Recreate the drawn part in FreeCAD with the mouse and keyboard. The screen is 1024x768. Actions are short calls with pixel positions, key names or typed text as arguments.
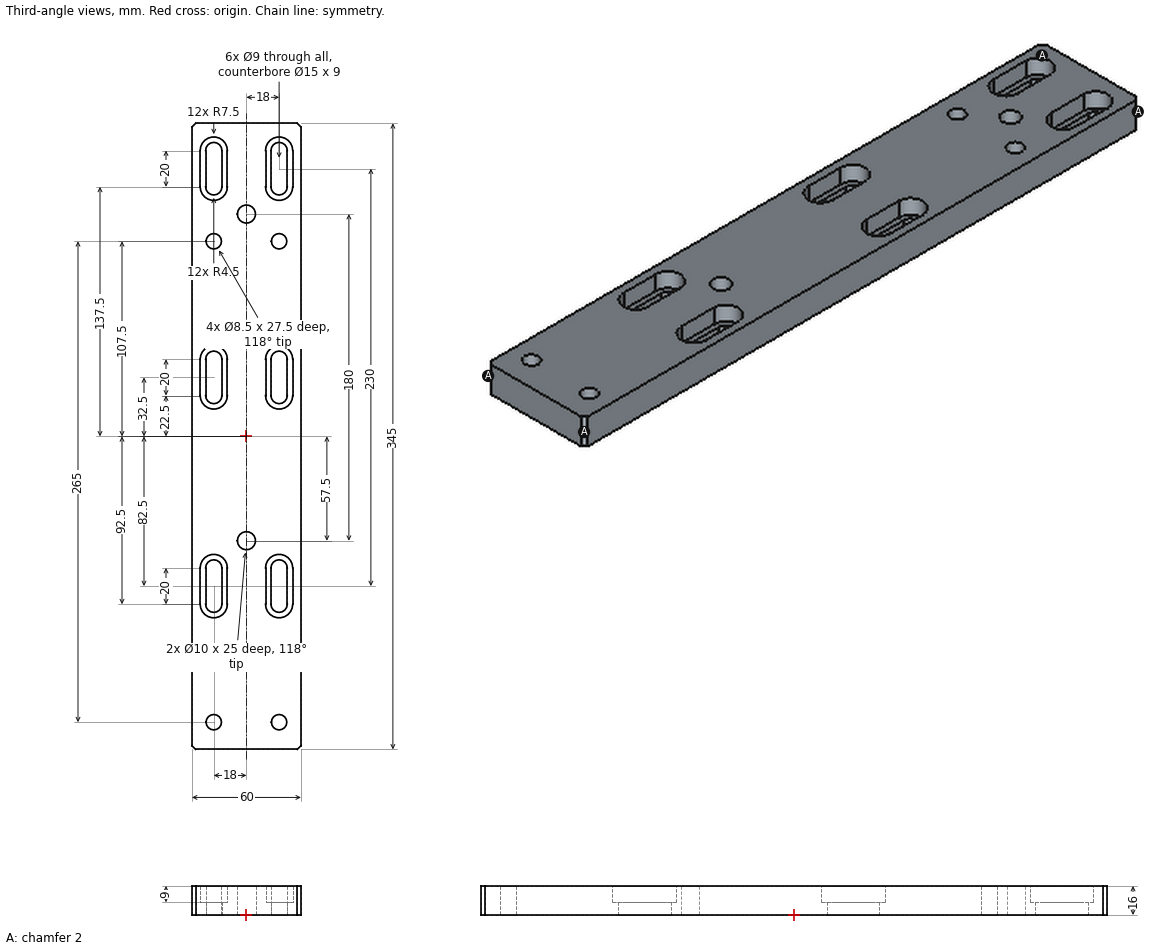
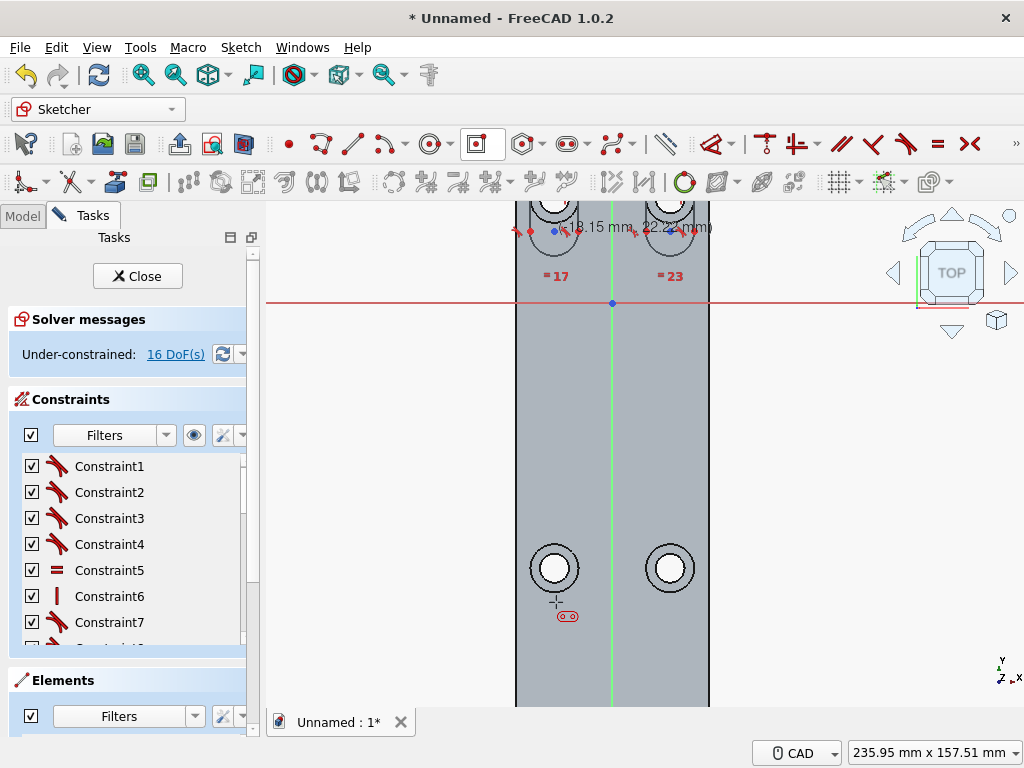
click(554, 600)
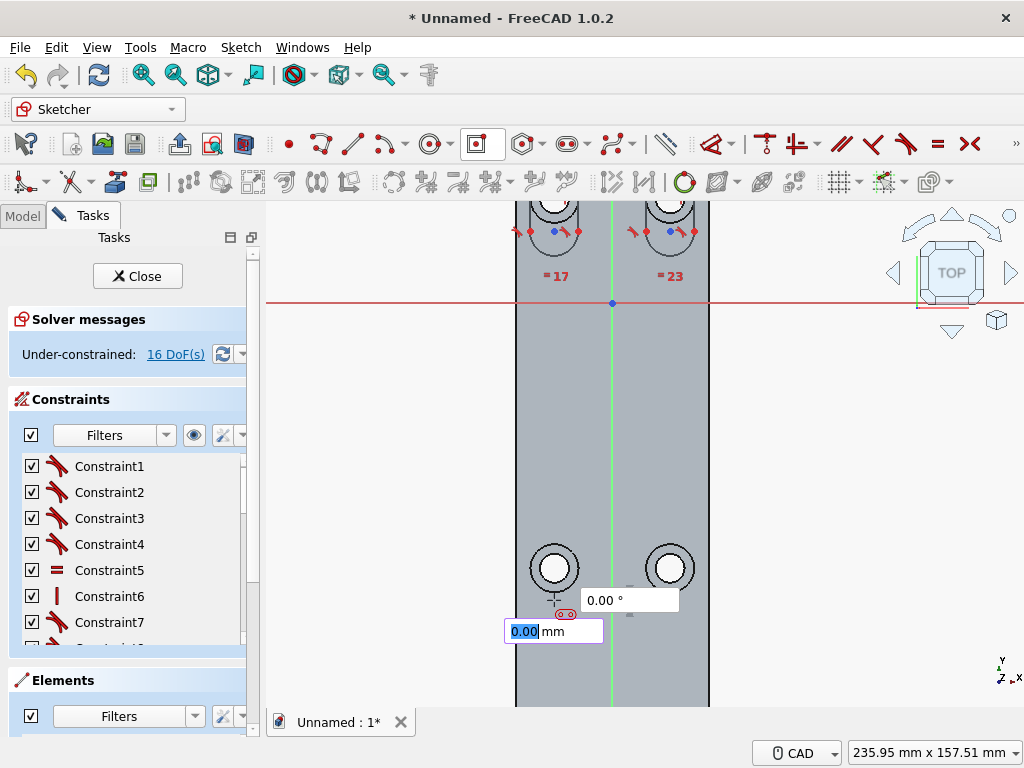
click(554, 536)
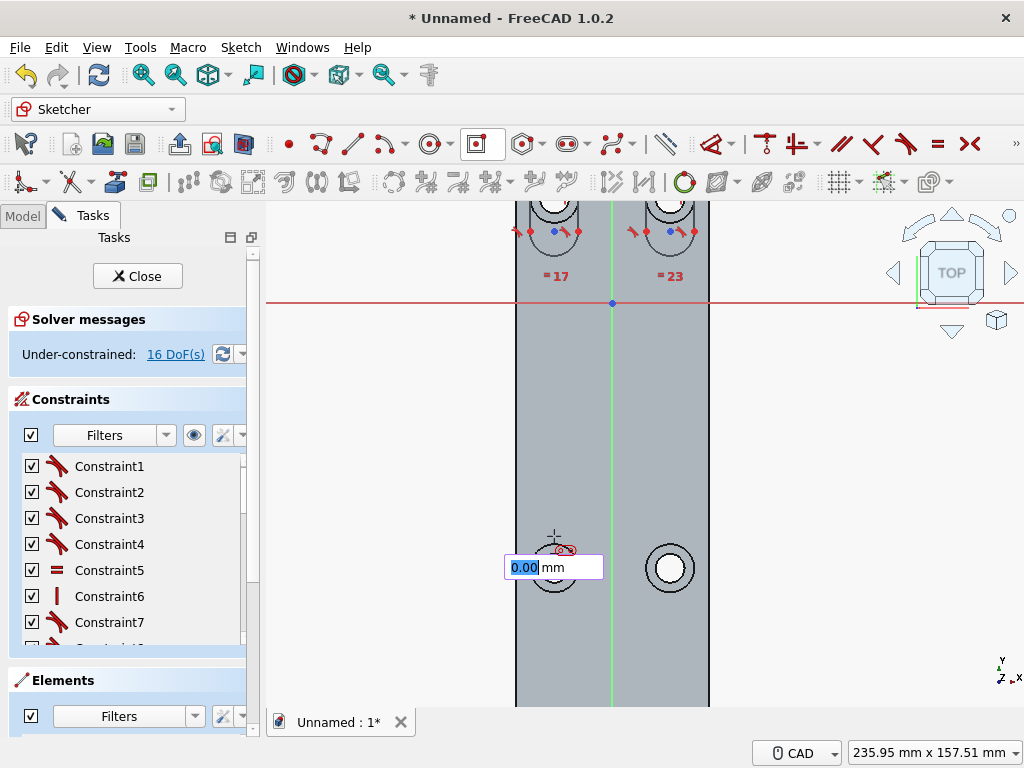
click(530, 568)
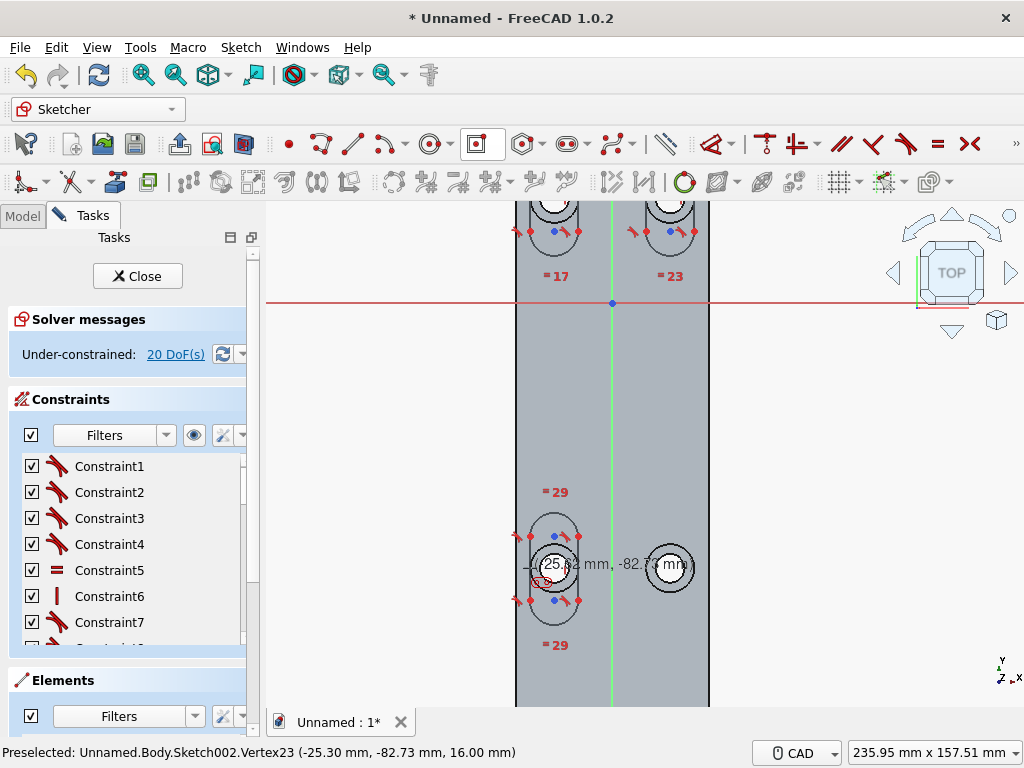
click(670, 600)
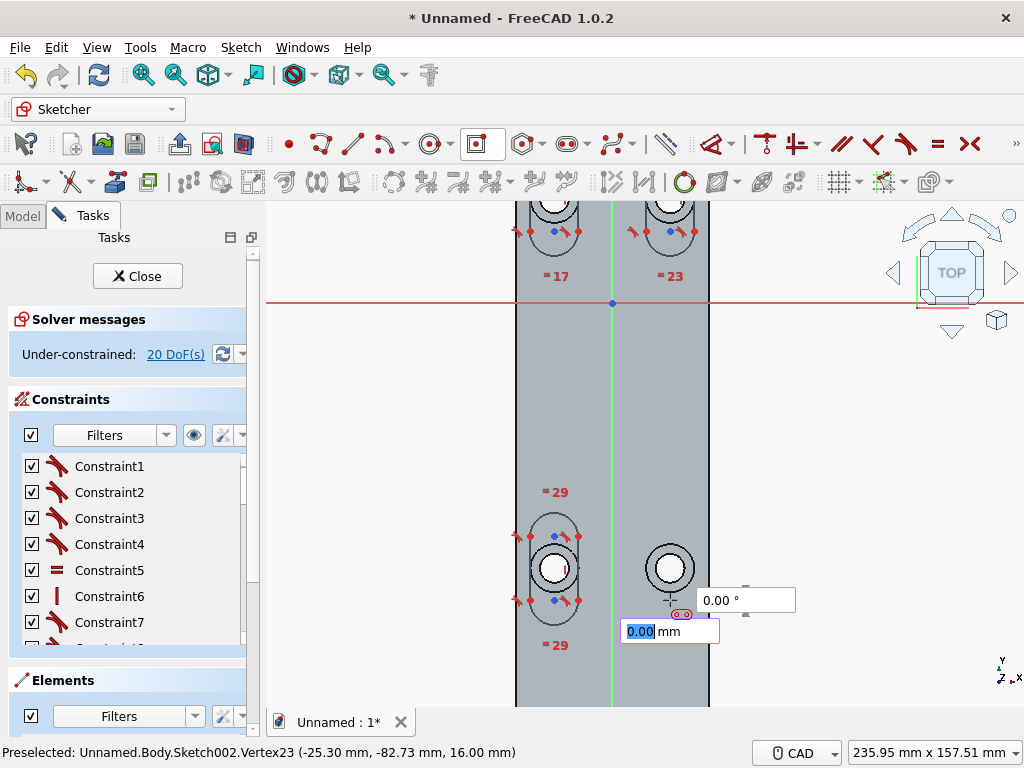
click(670, 536)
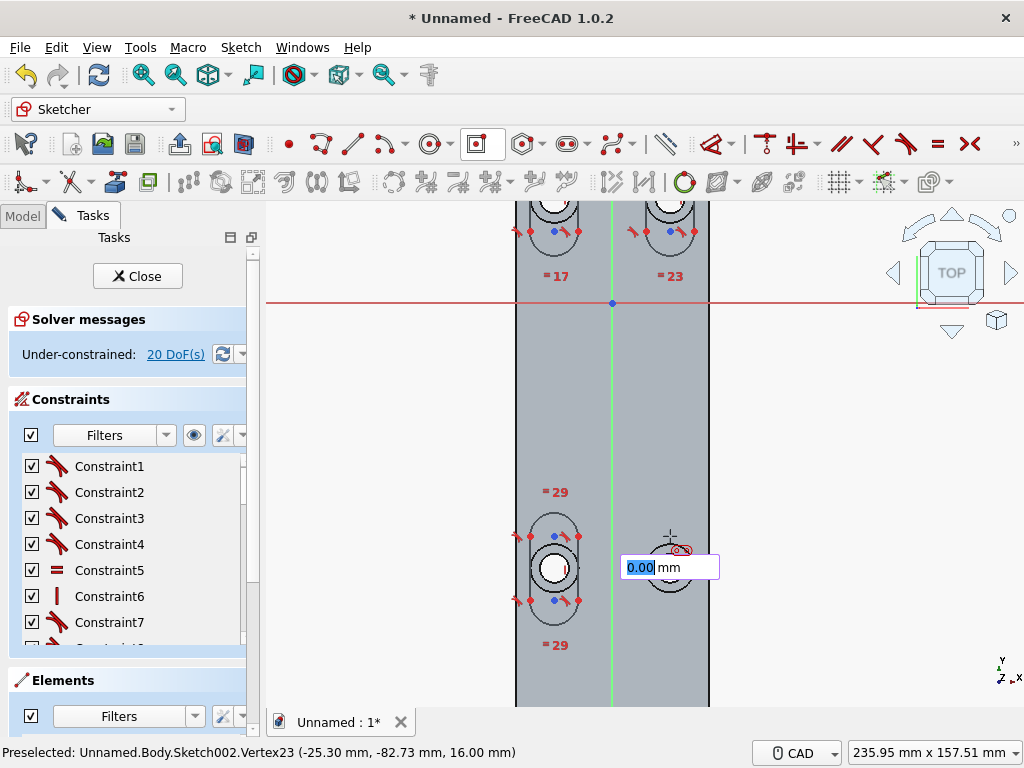
click(646, 568)
key(Escape)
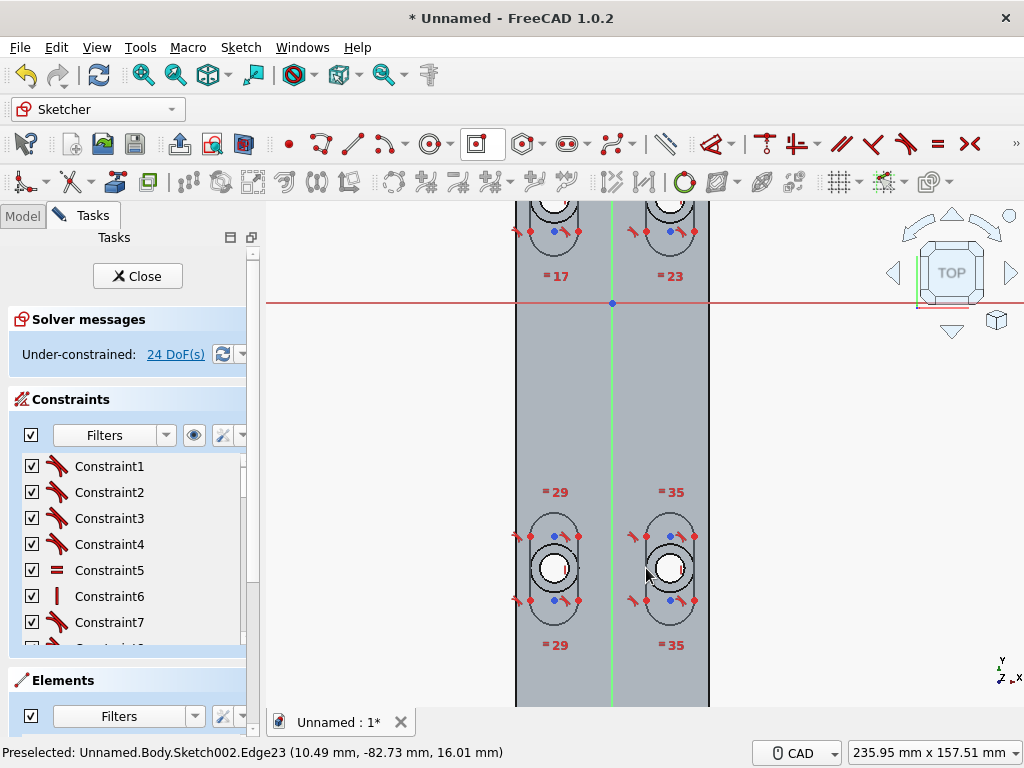
scroll(556, 602, down, 5)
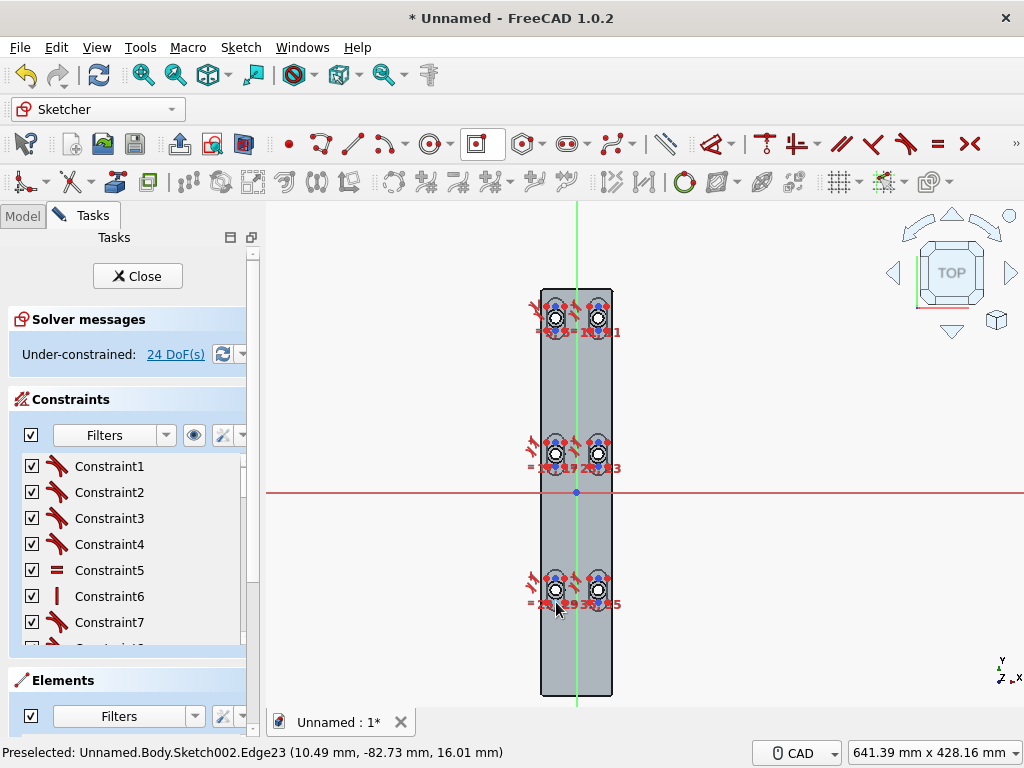
scroll(551, 338, up, 3)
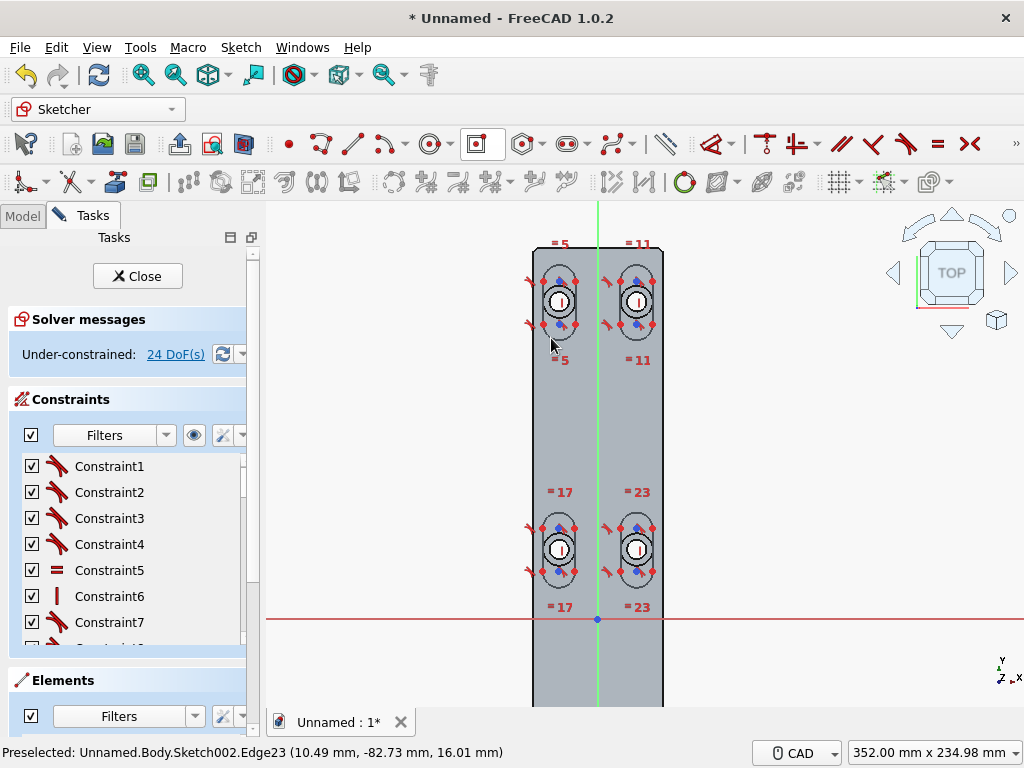
click(550, 337)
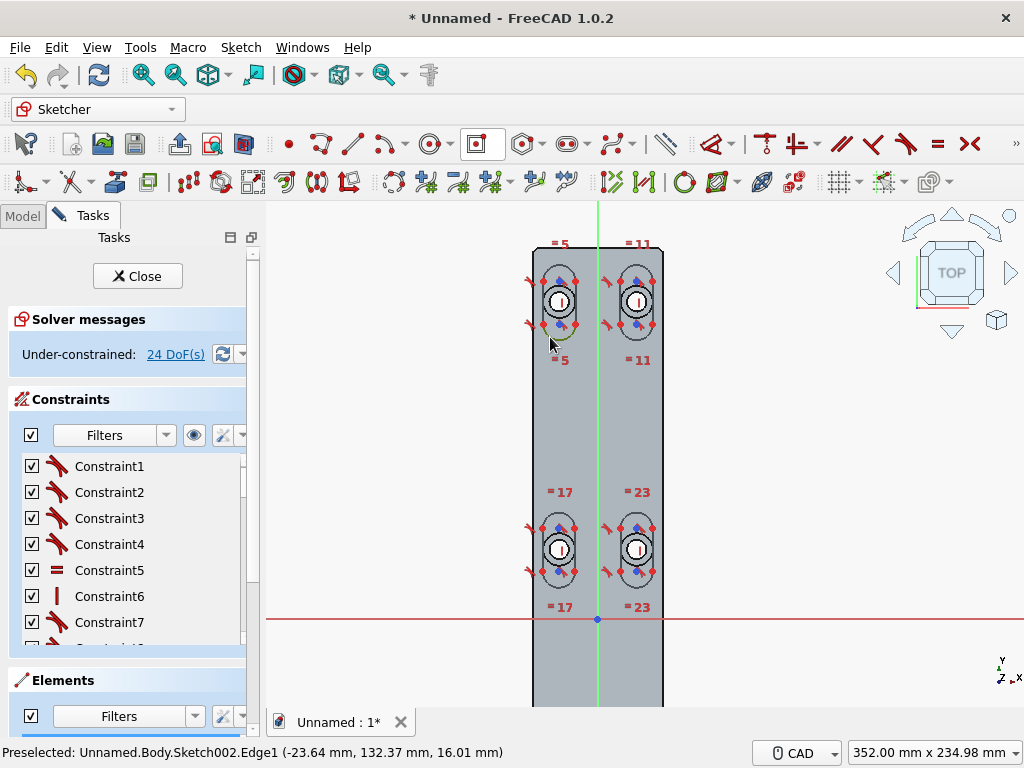
click(627, 337)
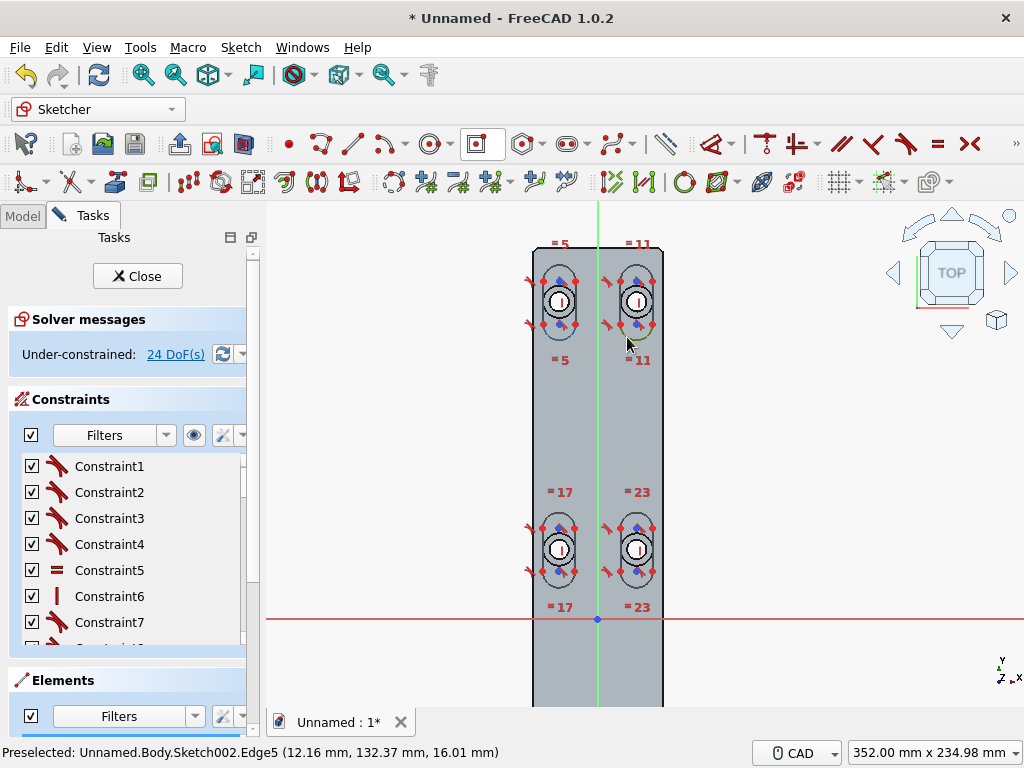
click(549, 585)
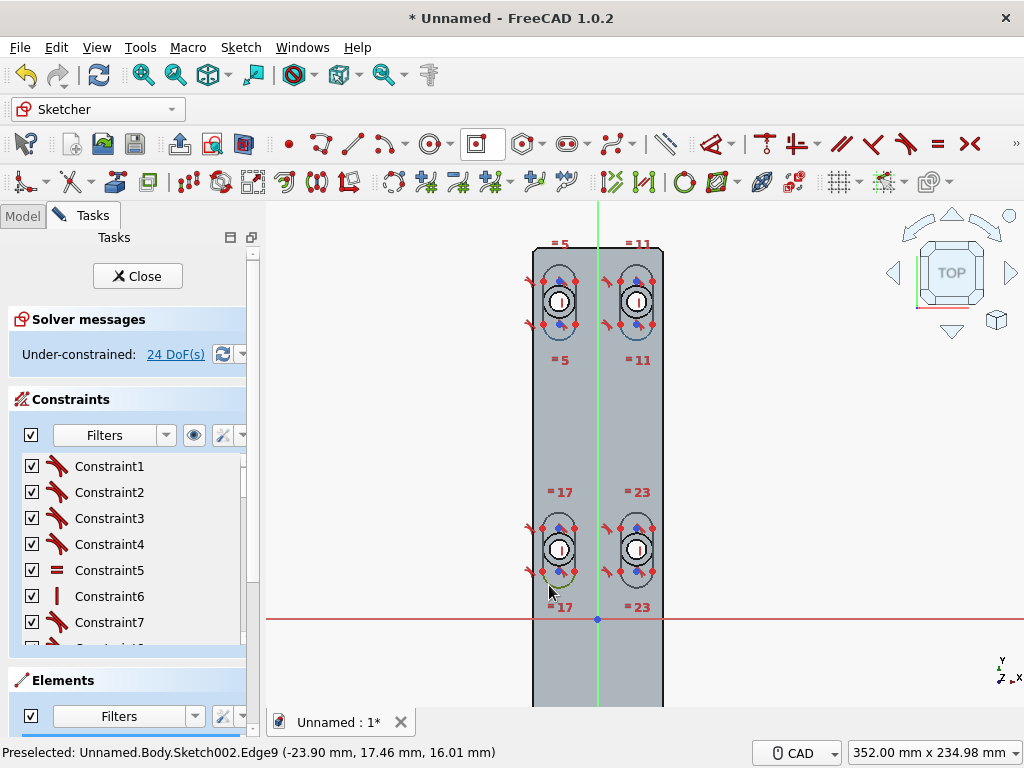
click(627, 585)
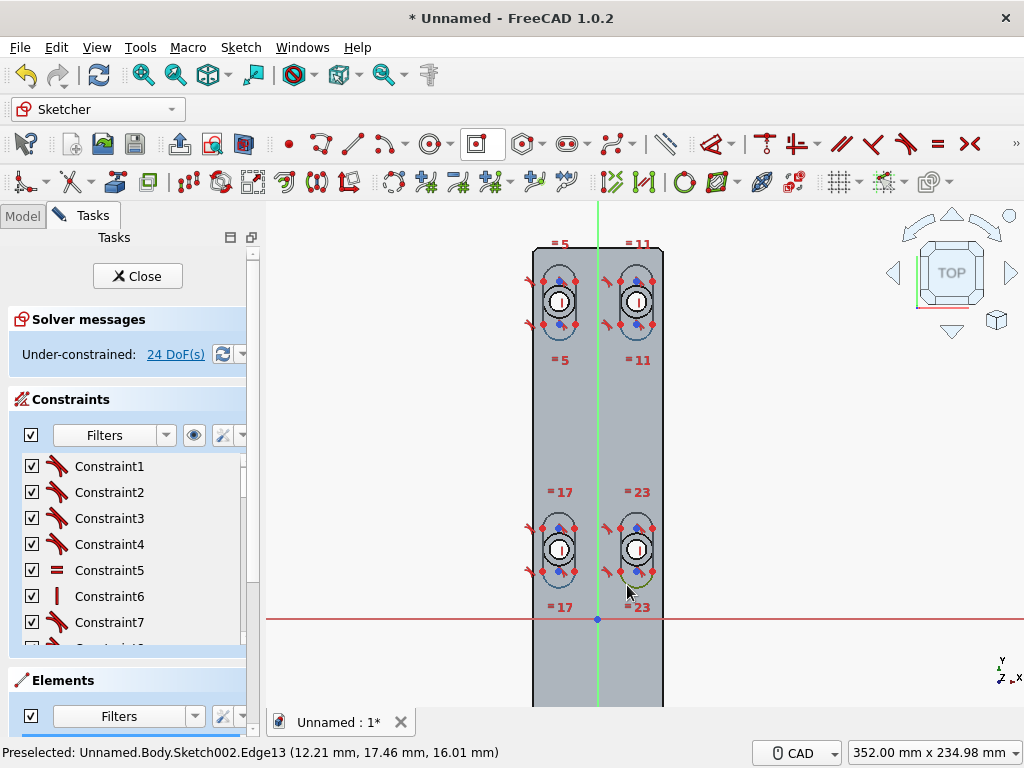
scroll(550, 338, down, 3)